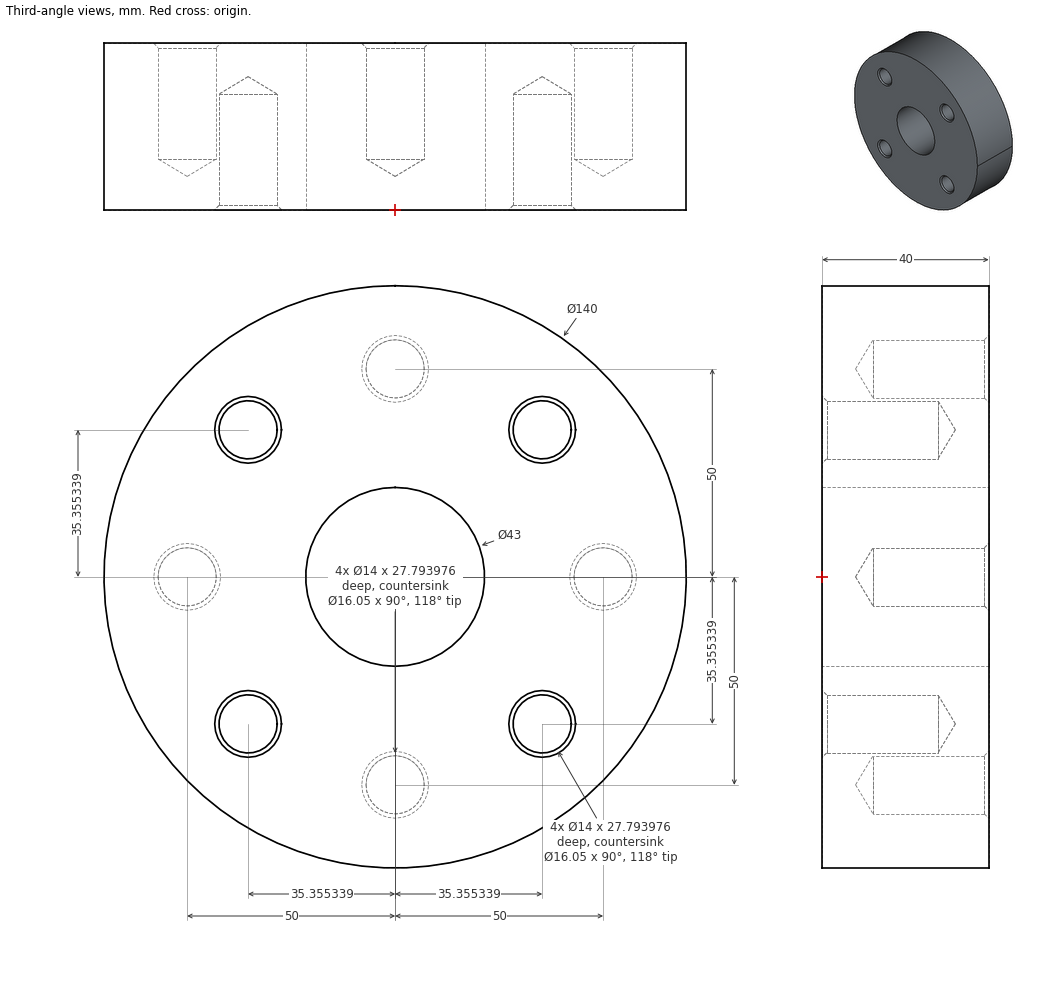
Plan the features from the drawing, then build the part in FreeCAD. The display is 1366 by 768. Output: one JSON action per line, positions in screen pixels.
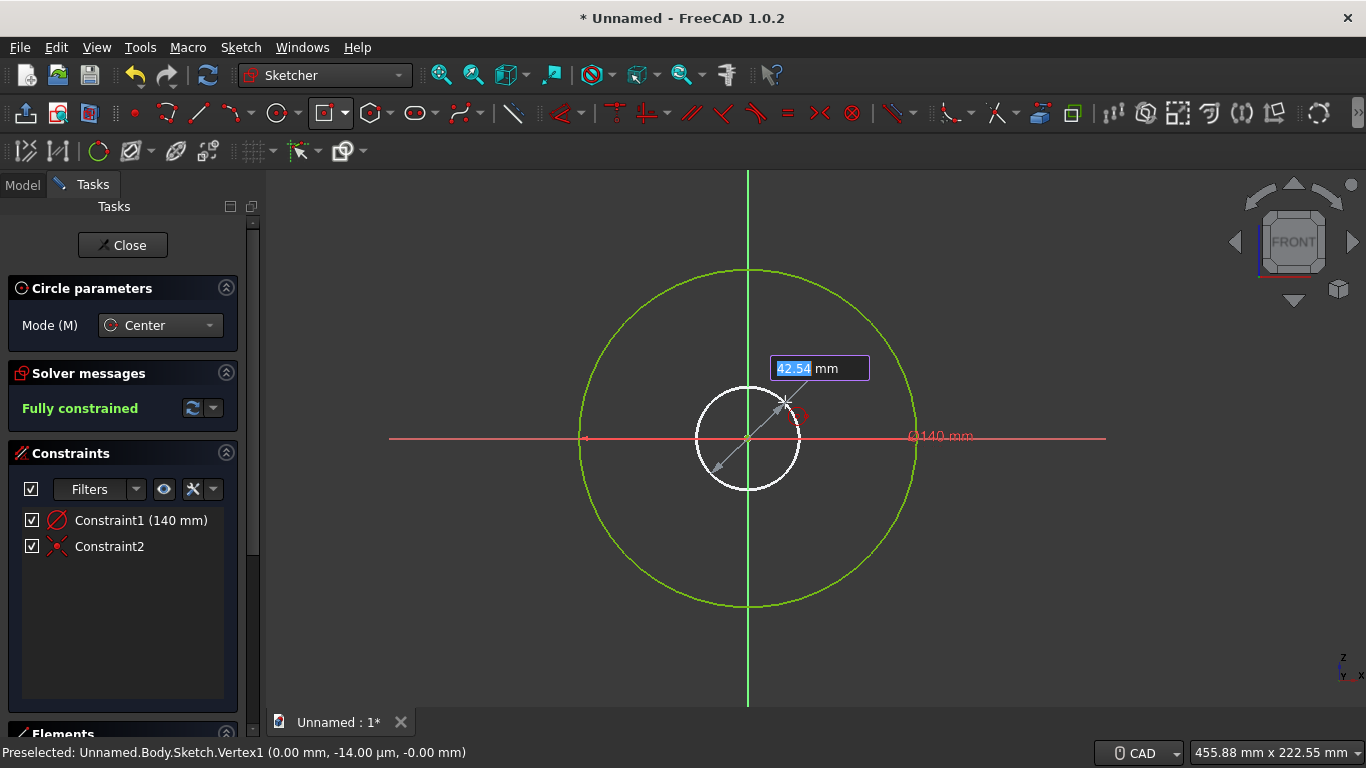
{"action": "type", "text": "43"}
{"action": "key", "text": "Return"}
{"action": "key", "text": "Escape"}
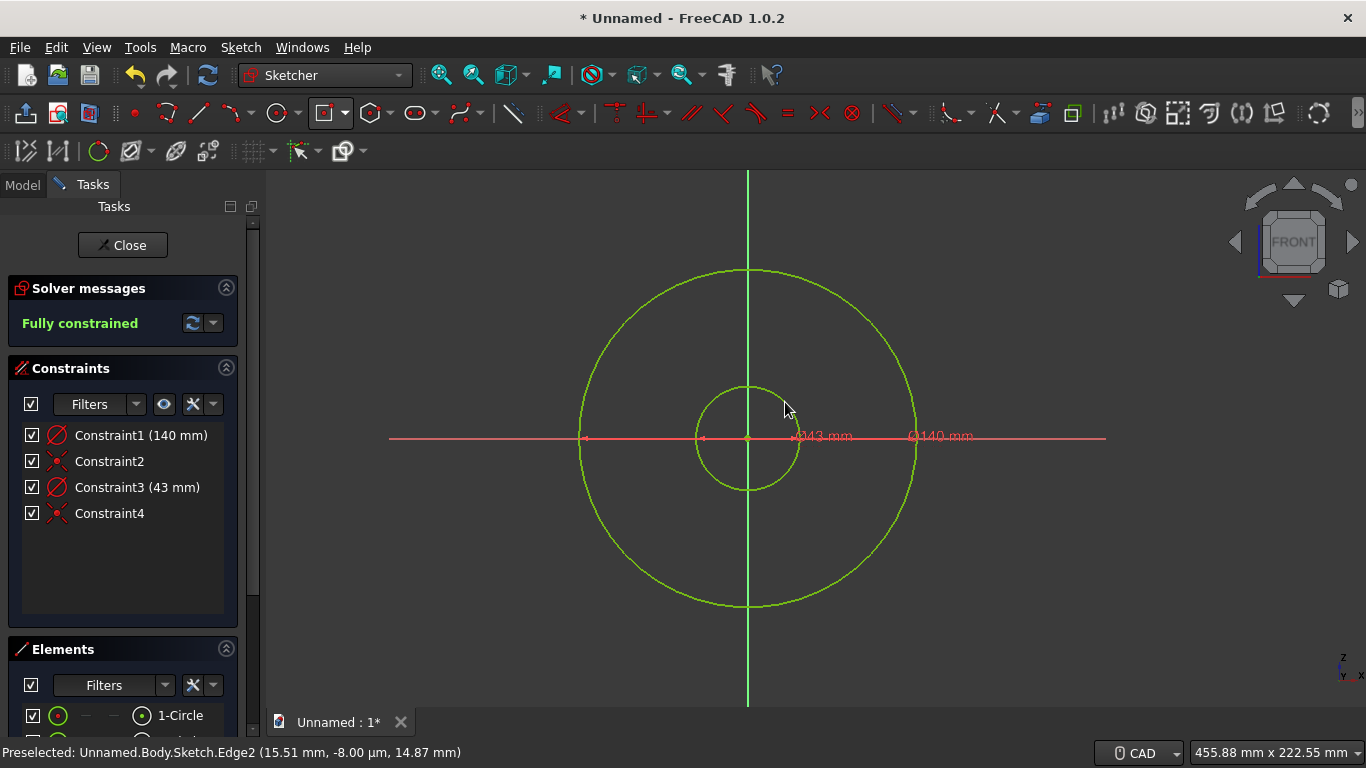
{"action": "left_click", "coordinate": [123, 245]}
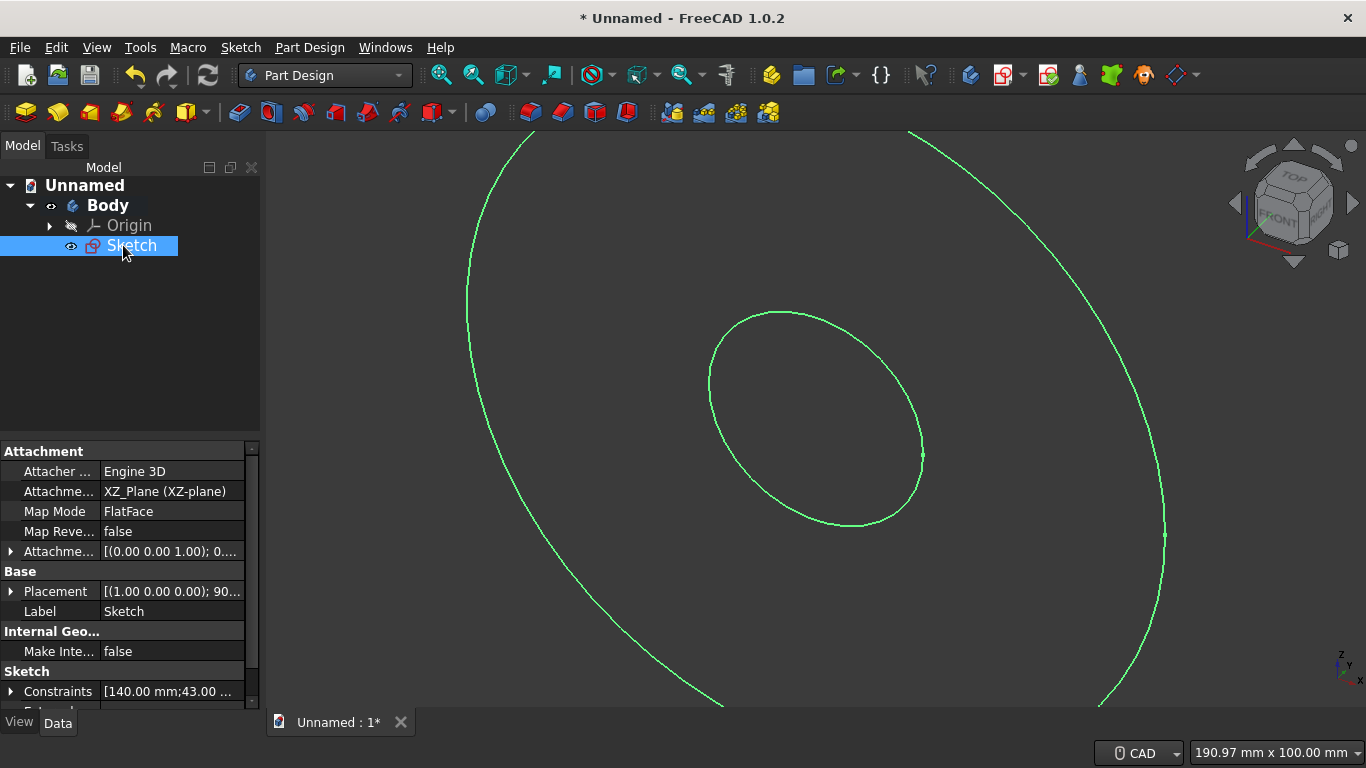
{"action": "left_click", "coordinate": [26, 112]}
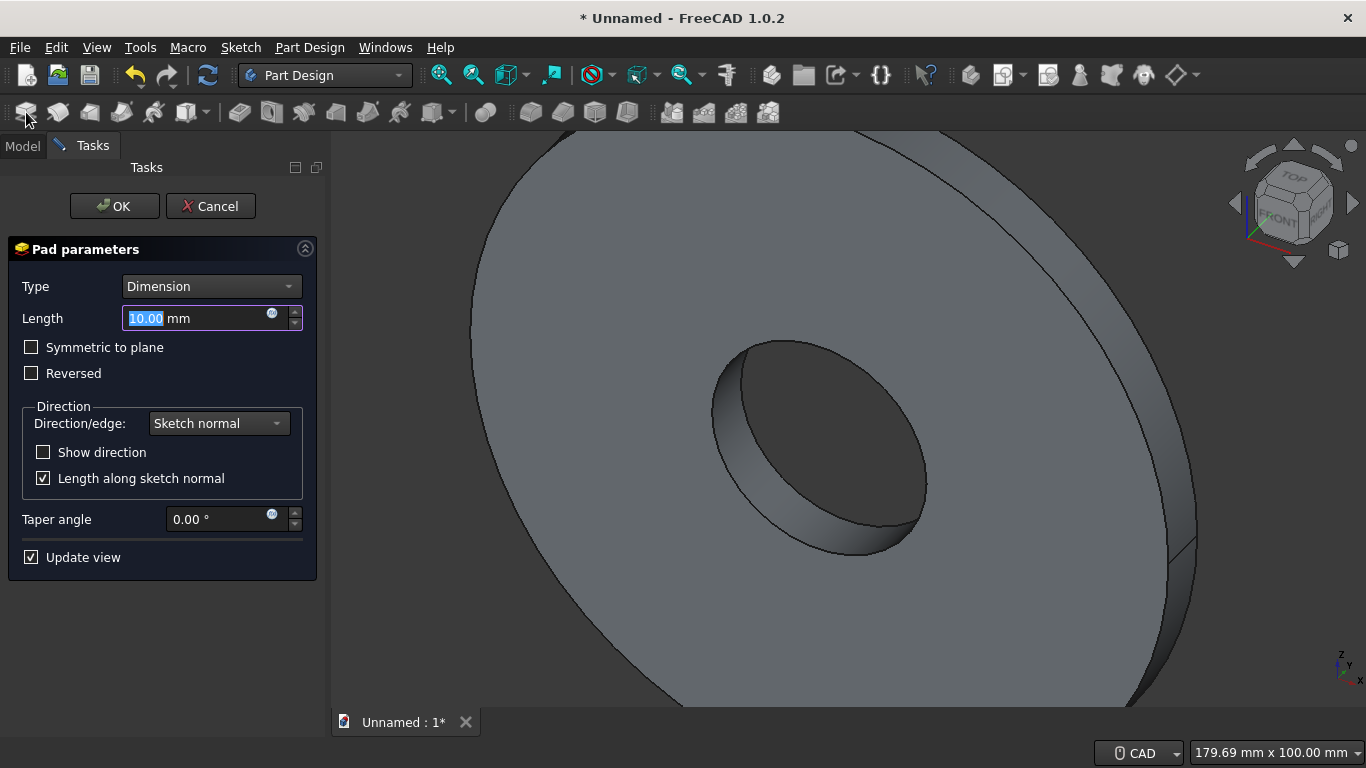
{"action": "type", "text": "40"}
{"action": "key", "text": "Tab"}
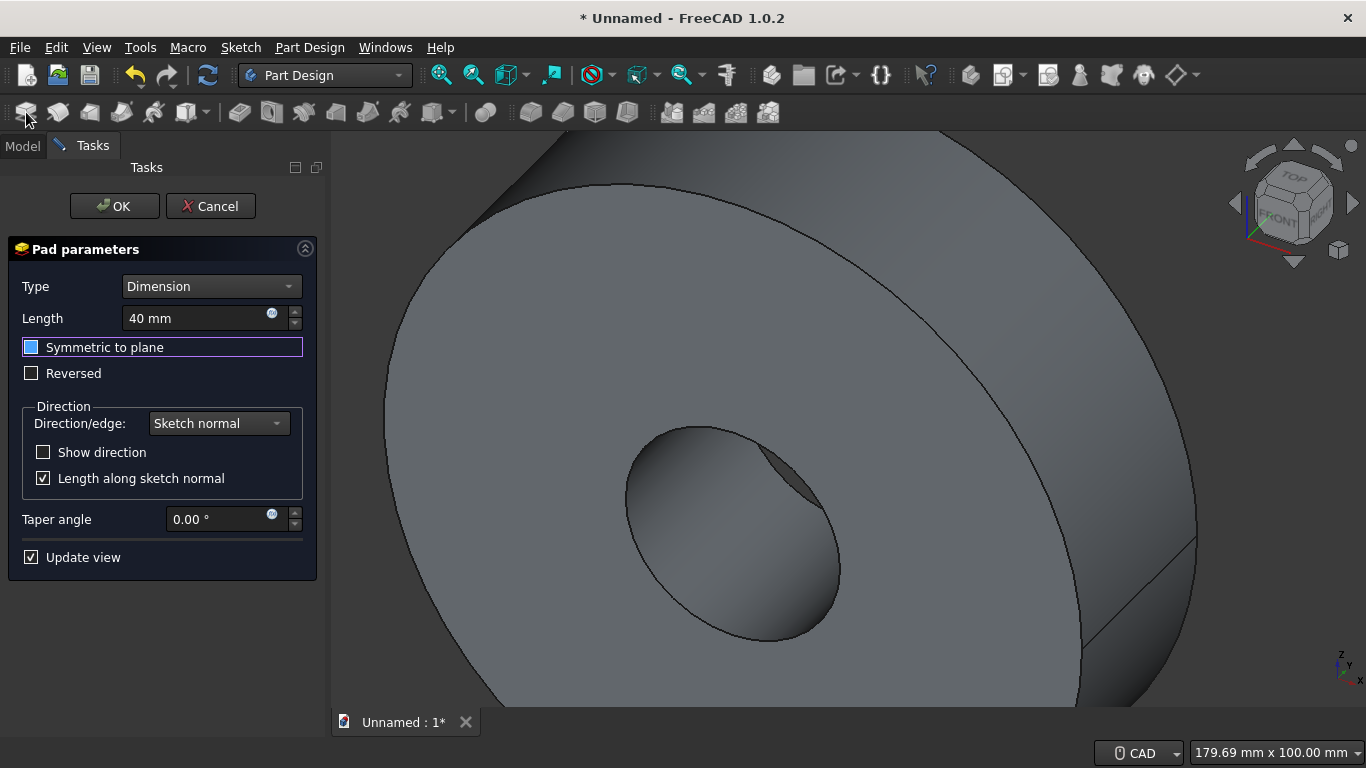
{"action": "left_click", "coordinate": [30, 373]}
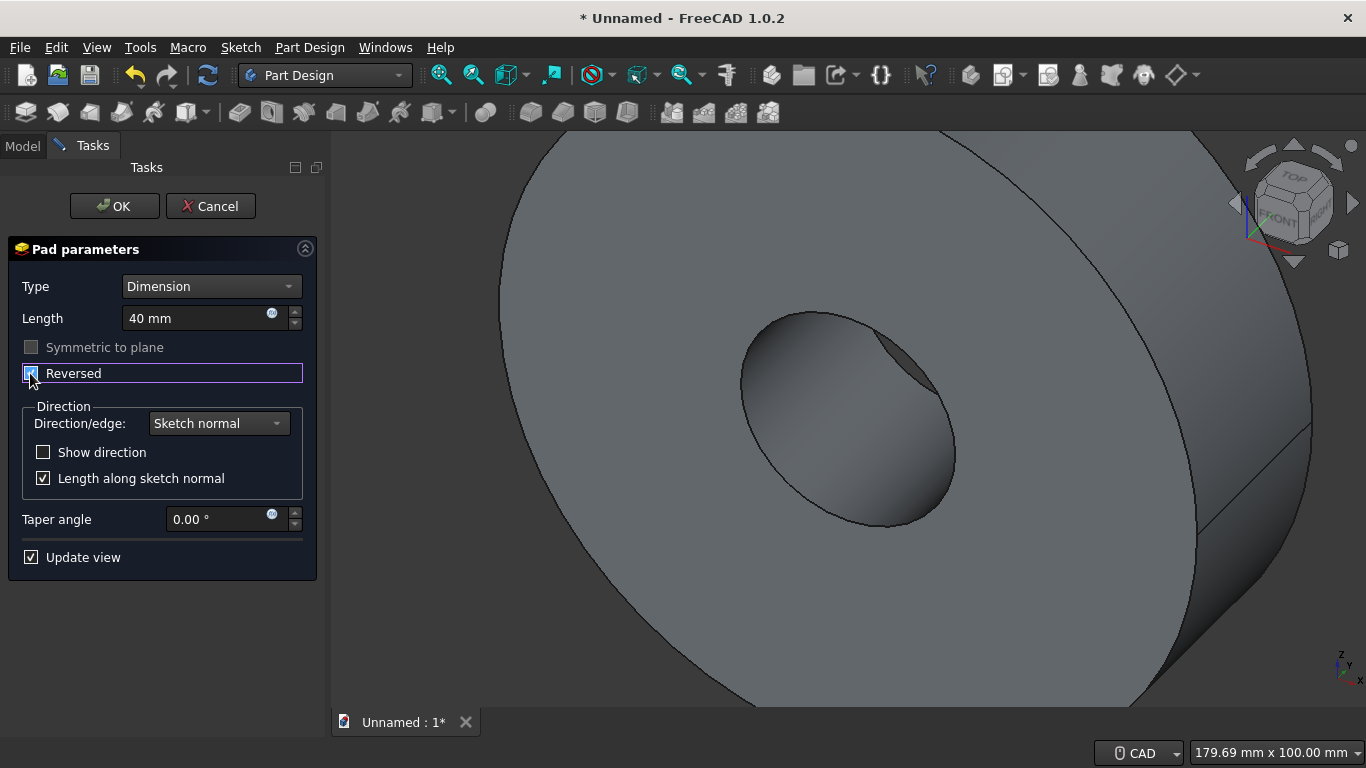
{"action": "left_click", "coordinate": [115, 206]}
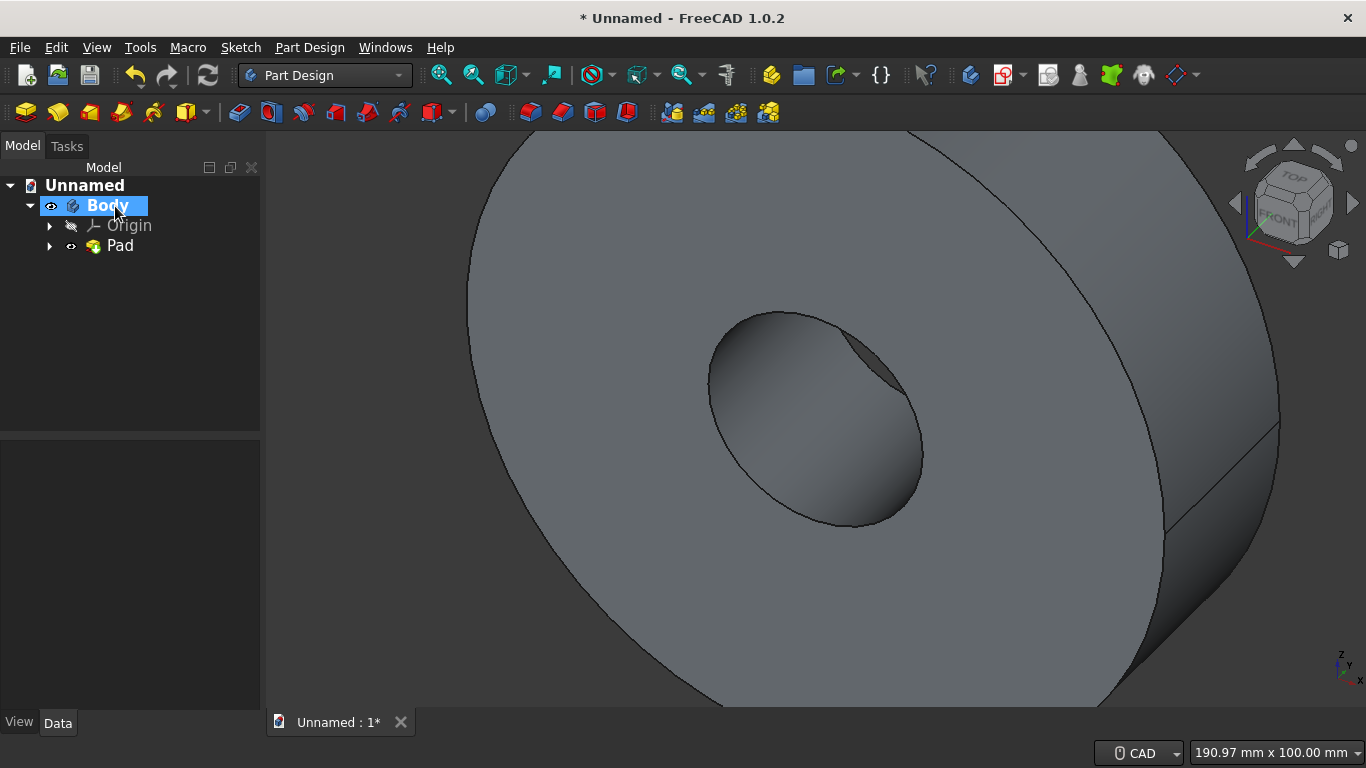
{"action": "left_click", "coordinate": [442, 76]}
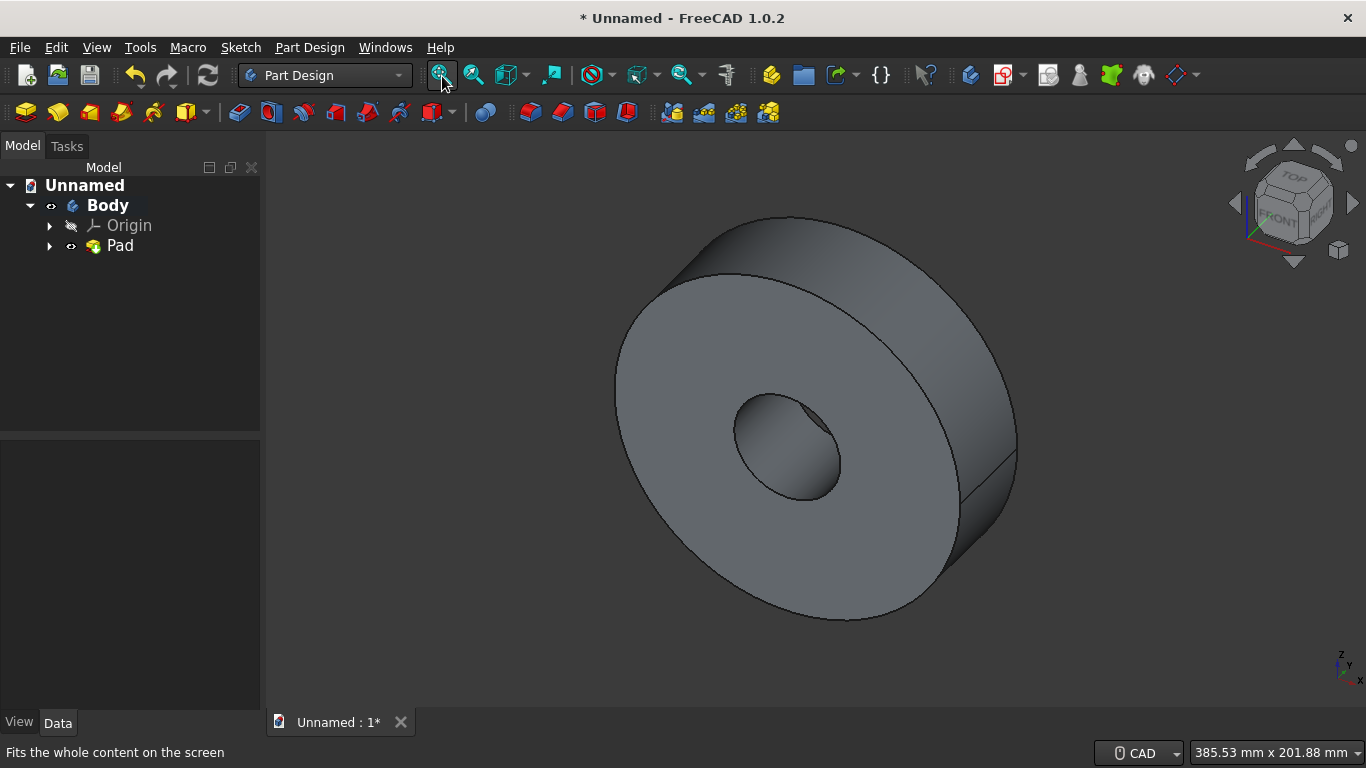
{"action": "key", "text": "4"}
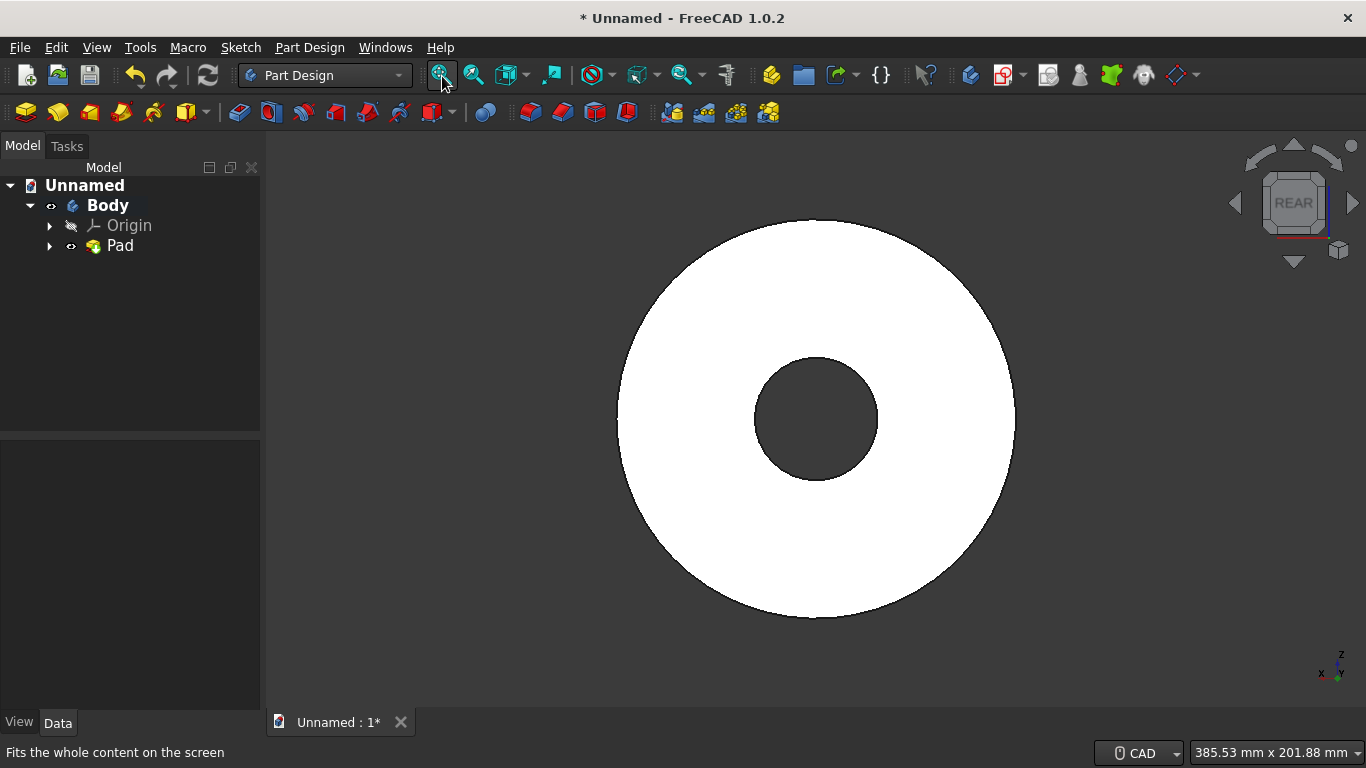
{"action": "left_click", "coordinate": [759, 304]}